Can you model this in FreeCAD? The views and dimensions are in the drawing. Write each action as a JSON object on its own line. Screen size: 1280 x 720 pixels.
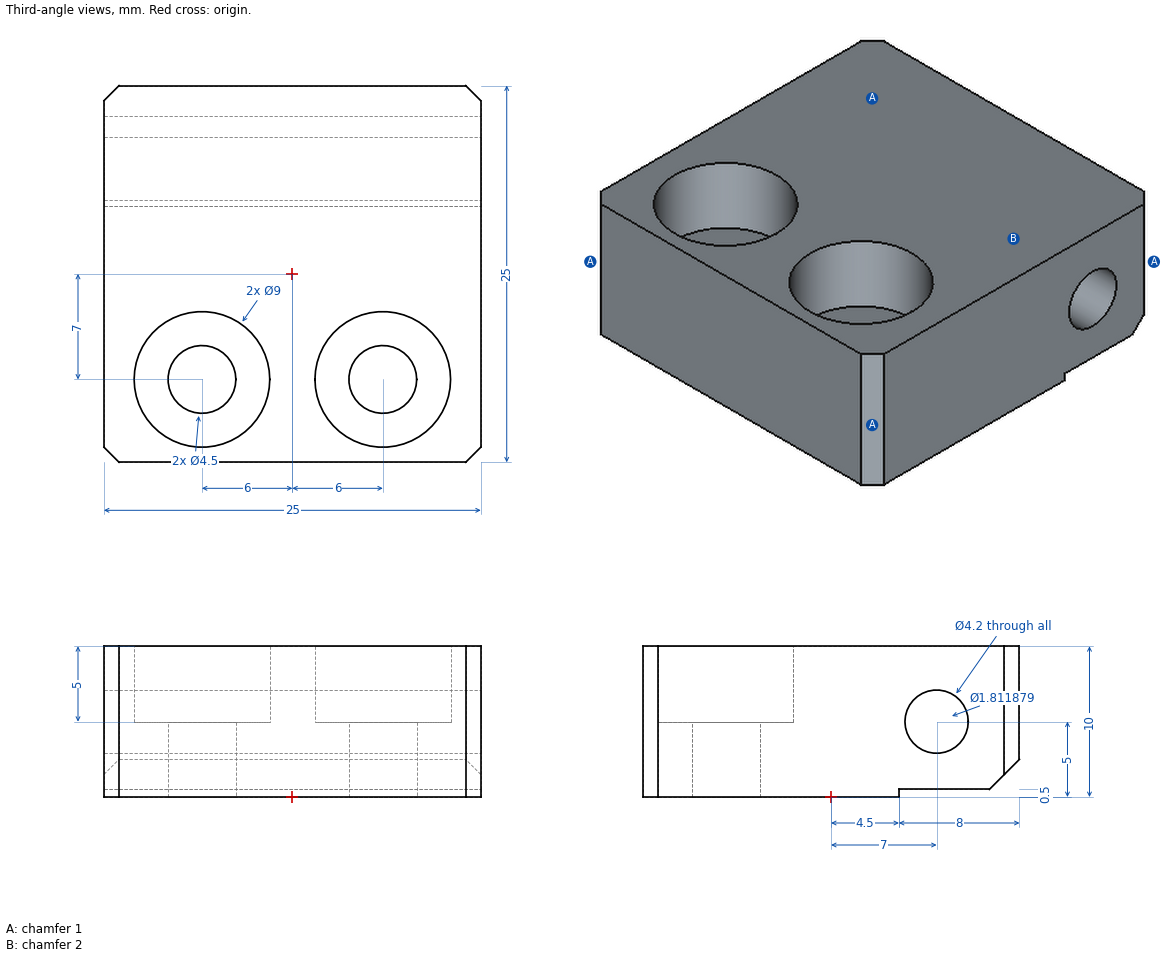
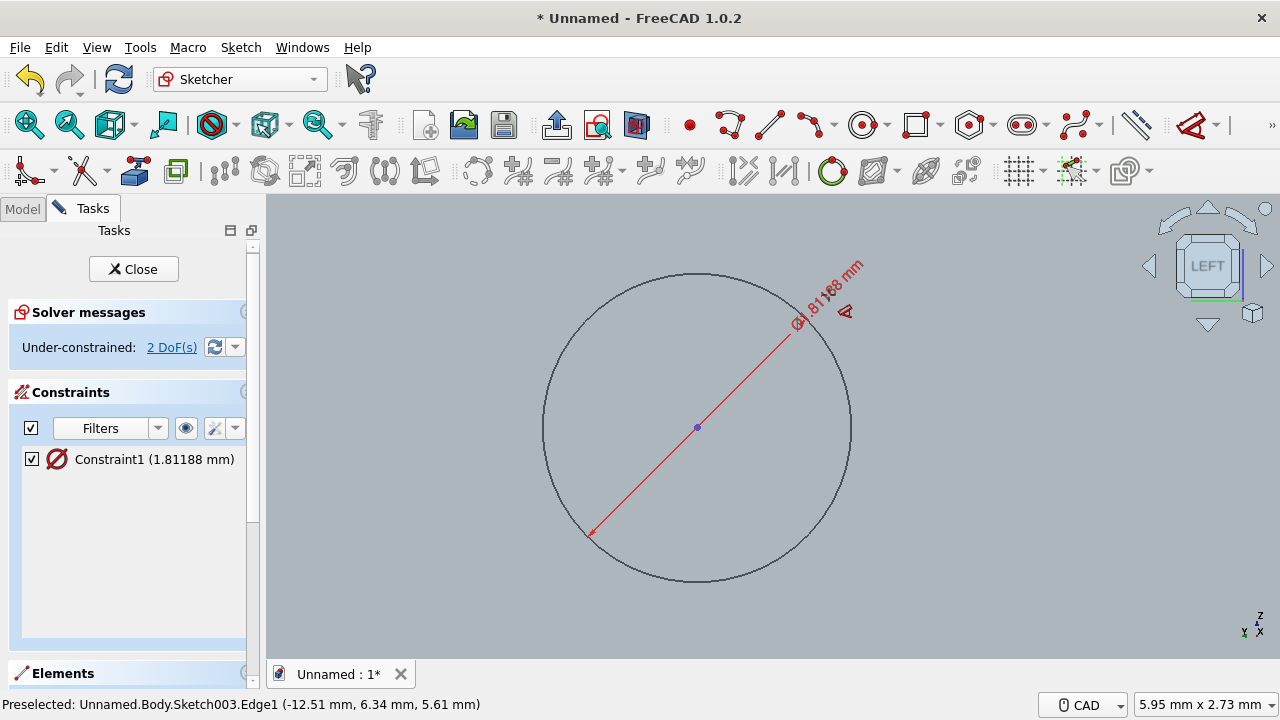
{"action": "left_click", "coordinate": [697, 428]}
{"action": "left_click", "coordinate": [906, 394]}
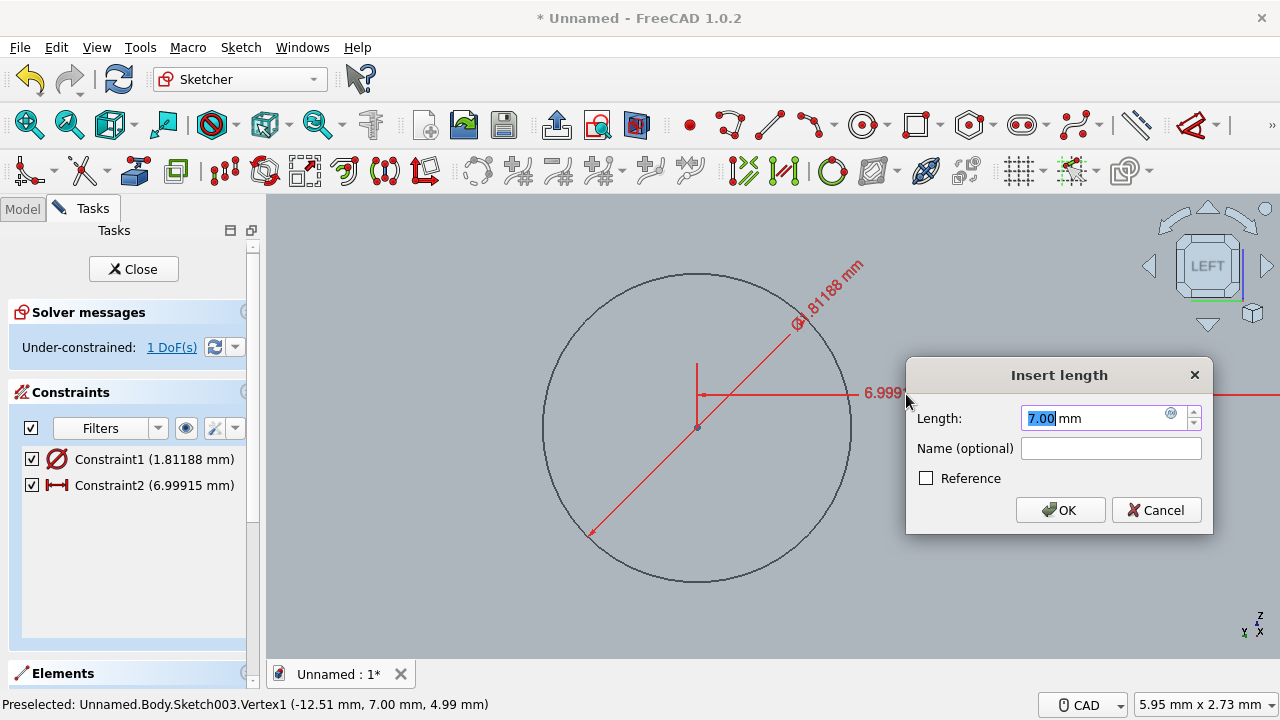
{"action": "type", "text": "7"}
{"action": "key", "text": "Return"}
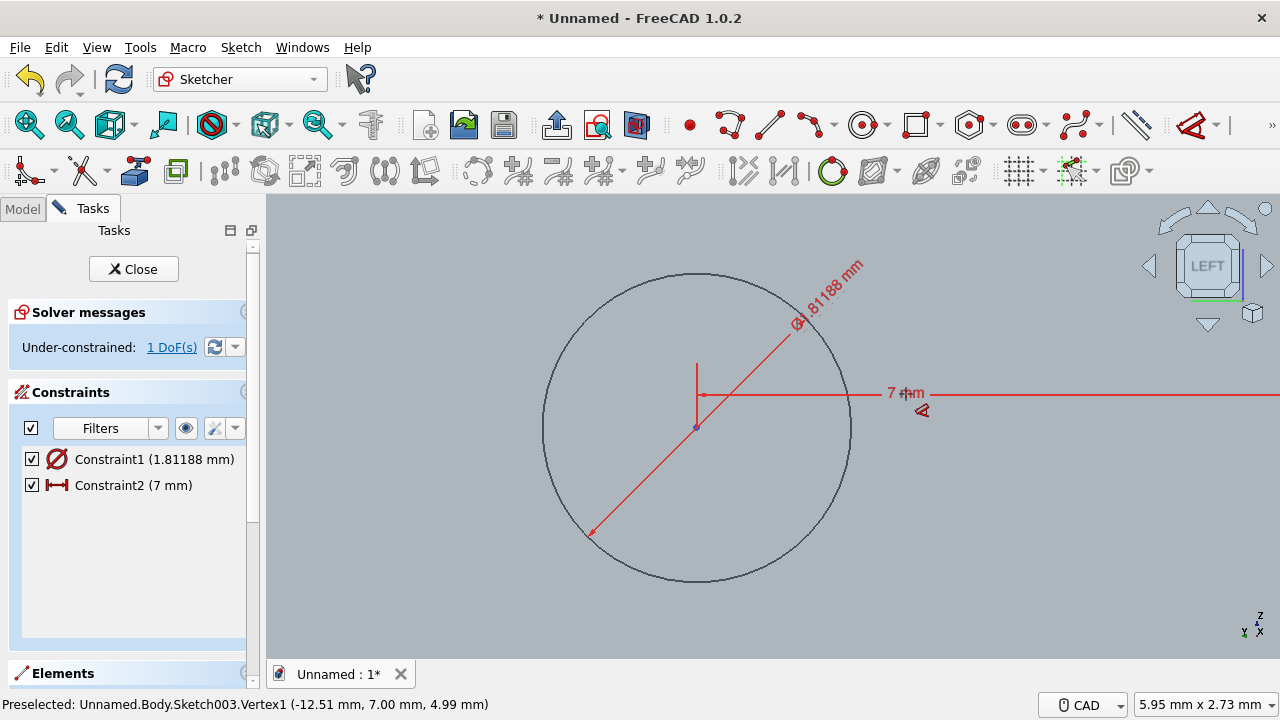
{"action": "left_click", "coordinate": [697, 428]}
{"action": "left_click", "coordinate": [663, 529]}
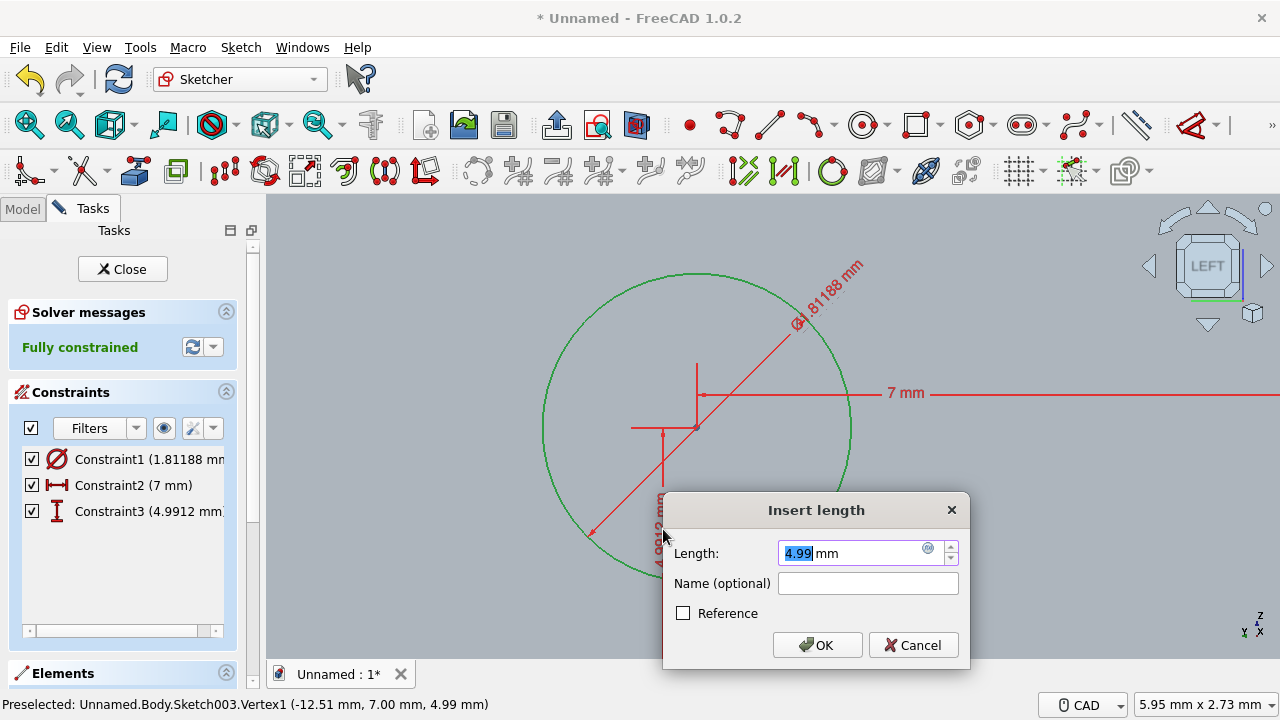
{"action": "type", "text": "5"}
{"action": "key", "text": "Return"}
{"action": "key", "text": "Escape"}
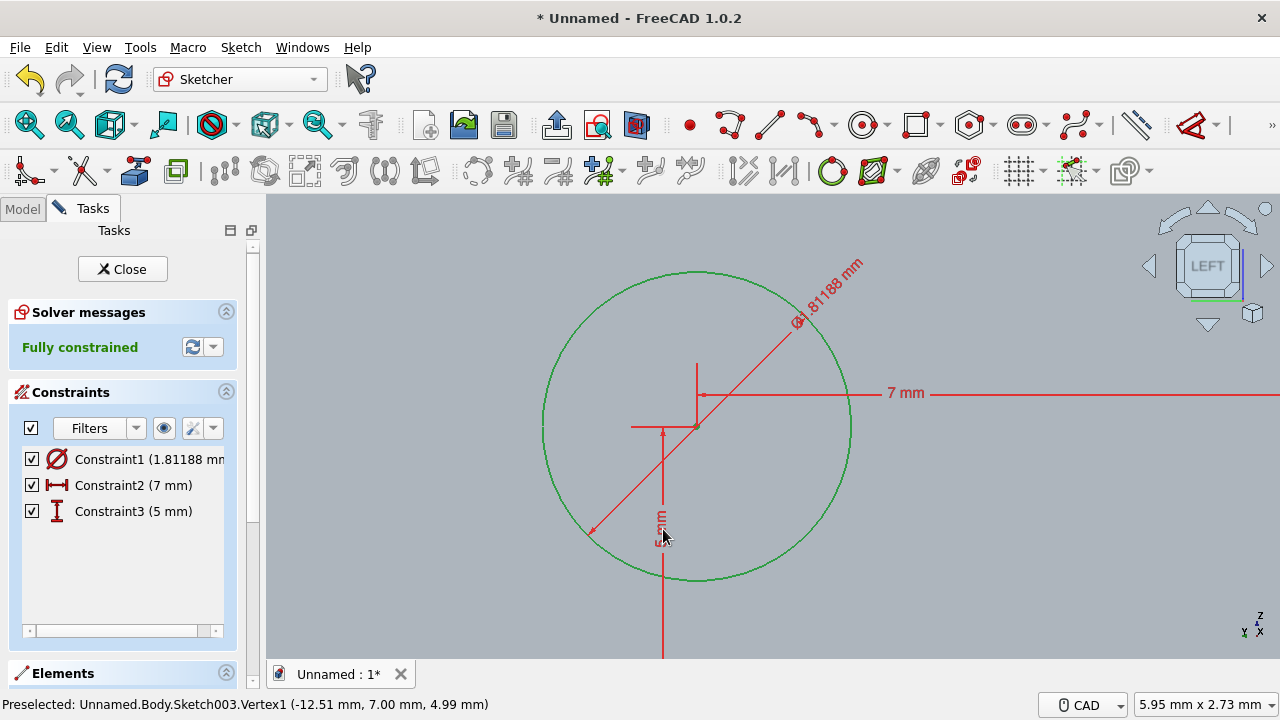
{"action": "left_click", "coordinate": [123, 269]}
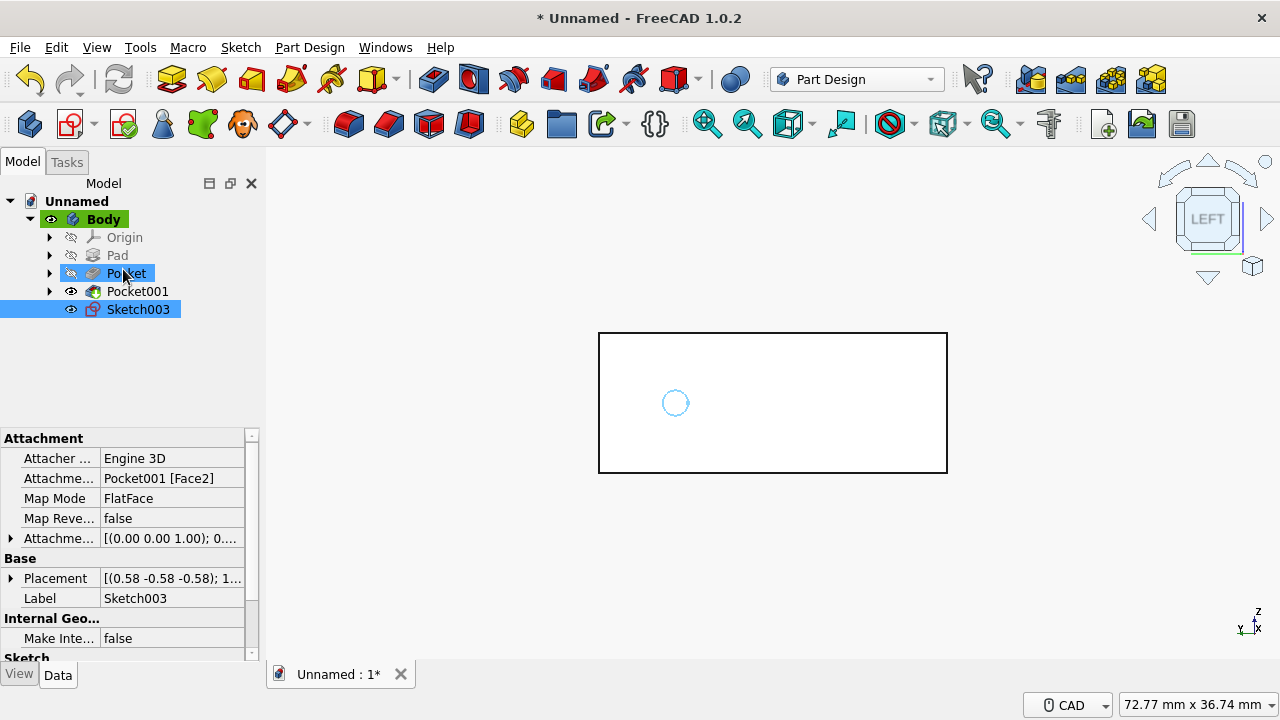
{"action": "left_click", "coordinate": [434, 80]}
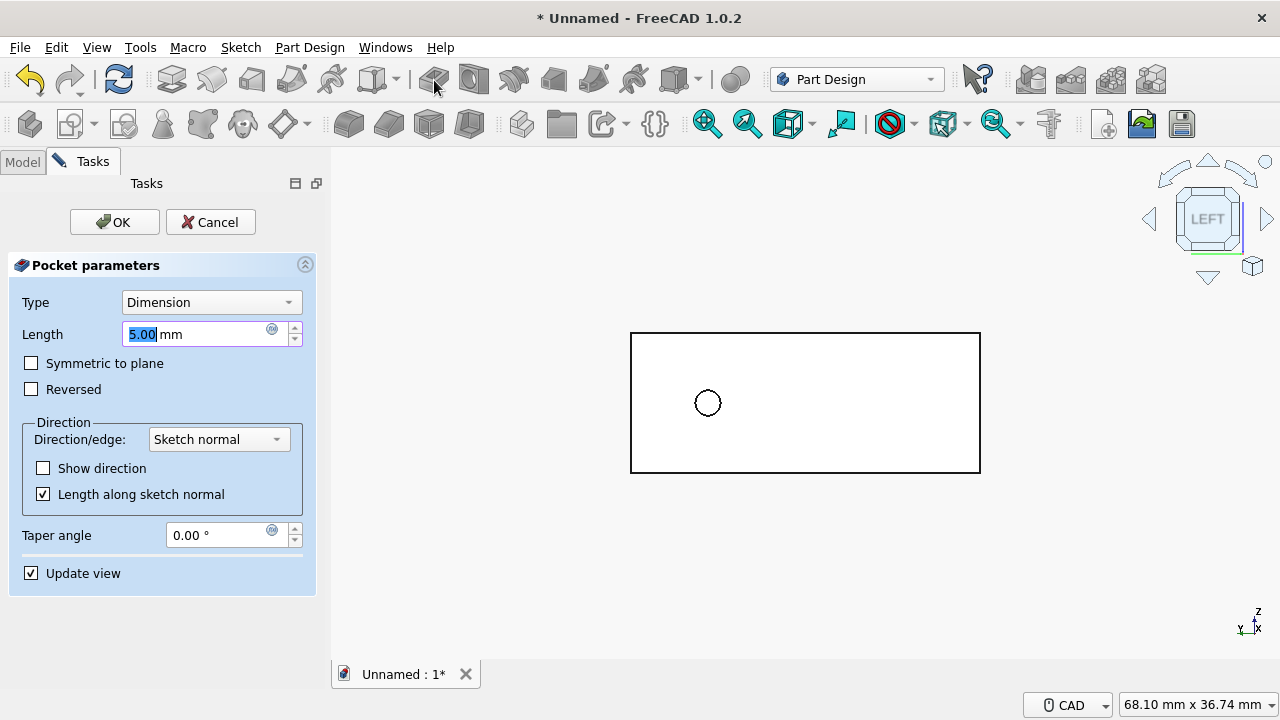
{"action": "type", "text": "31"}
{"action": "key", "text": "Tab"}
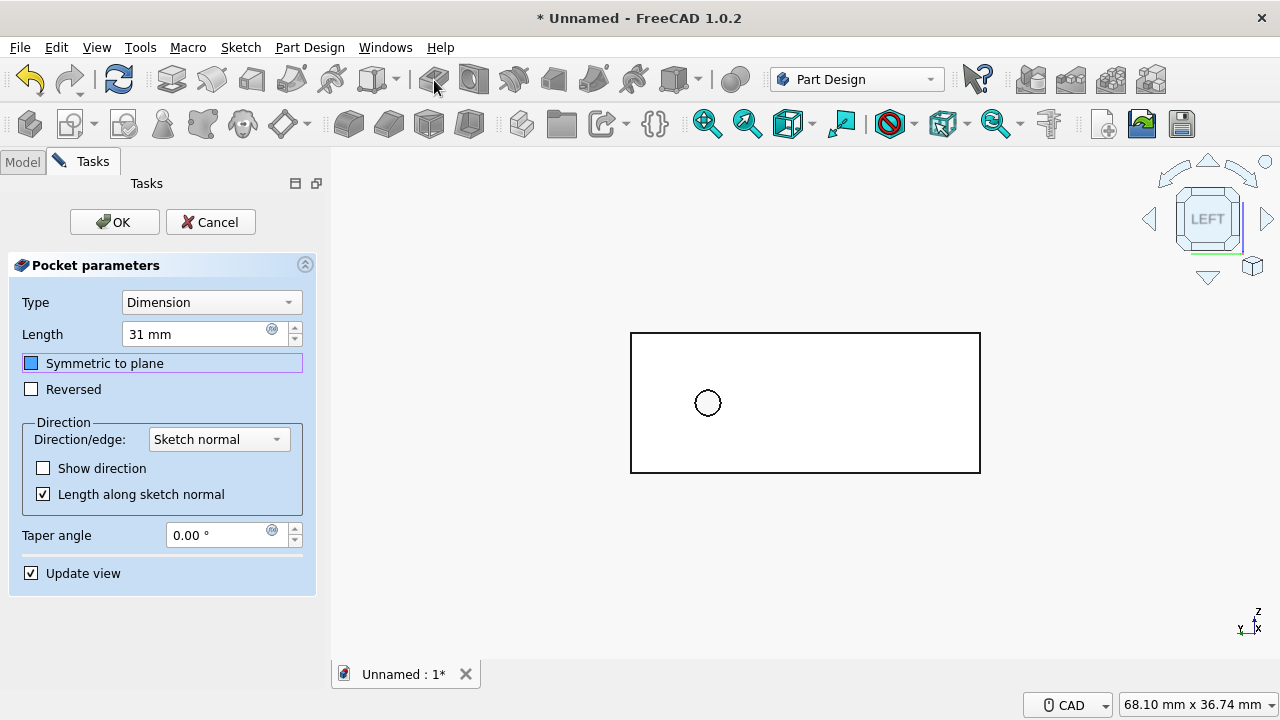
{"action": "left_click", "coordinate": [115, 222]}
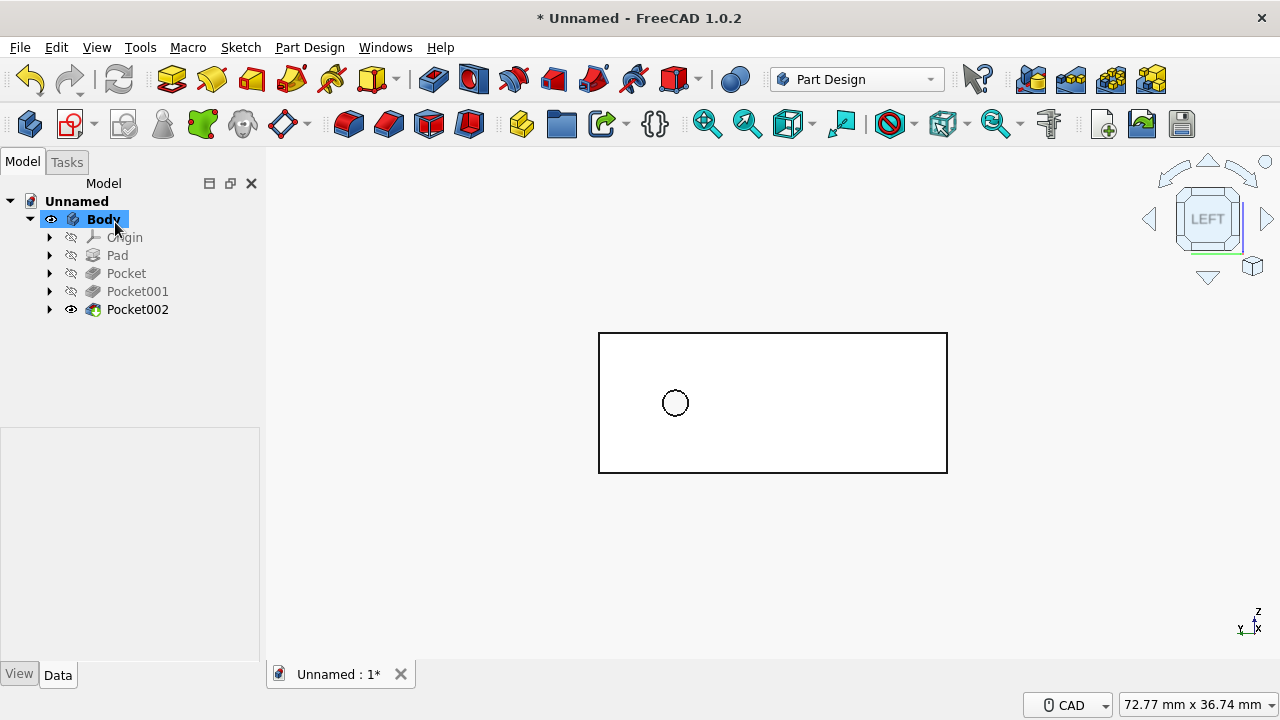
{"action": "key", "text": "v f"}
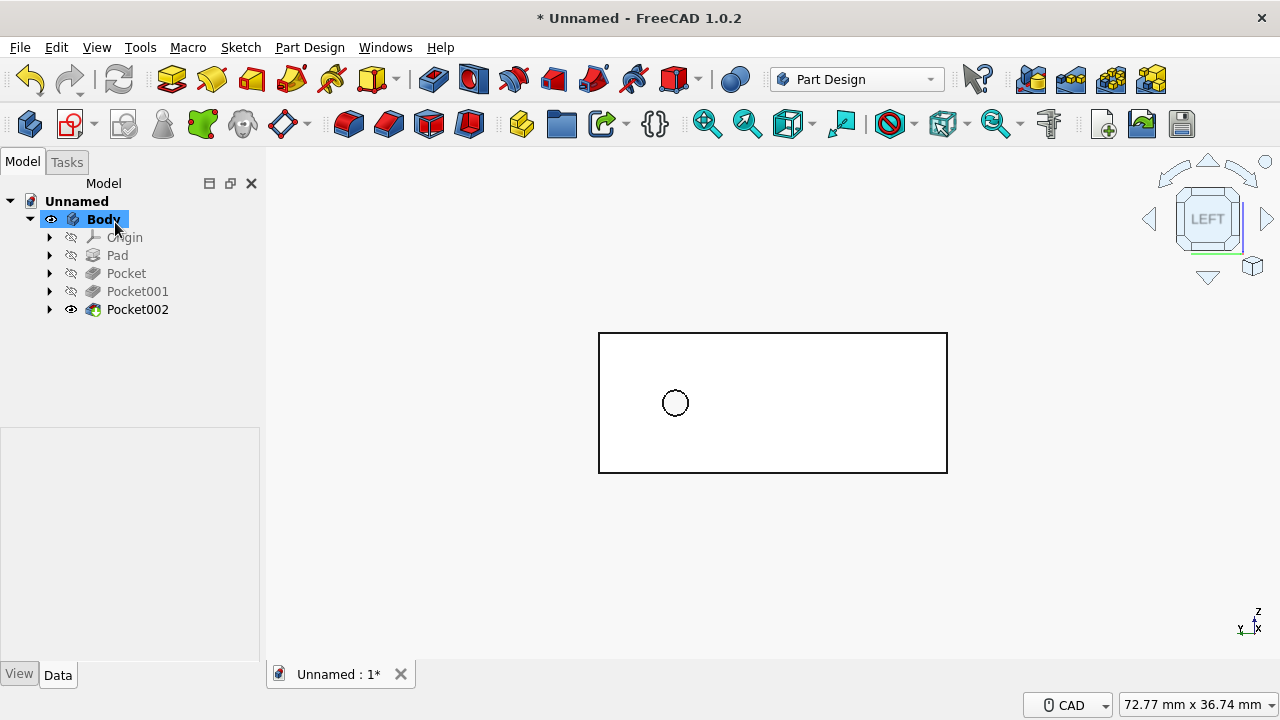
{"action": "left_click", "coordinate": [773, 402]}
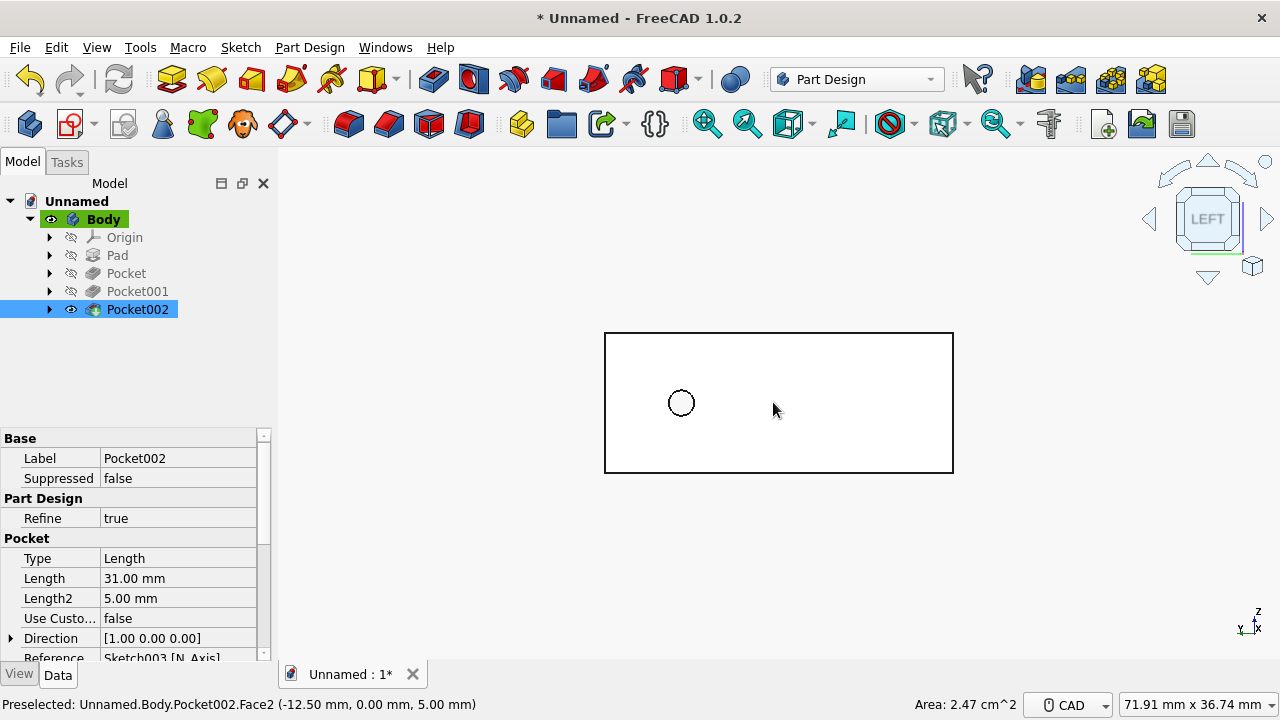
{"action": "left_click", "coordinate": [70, 124]}